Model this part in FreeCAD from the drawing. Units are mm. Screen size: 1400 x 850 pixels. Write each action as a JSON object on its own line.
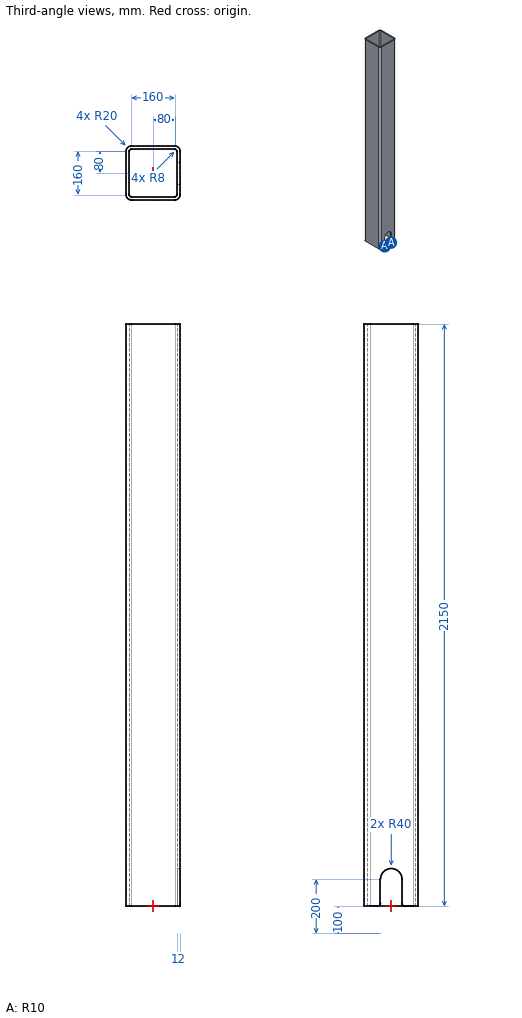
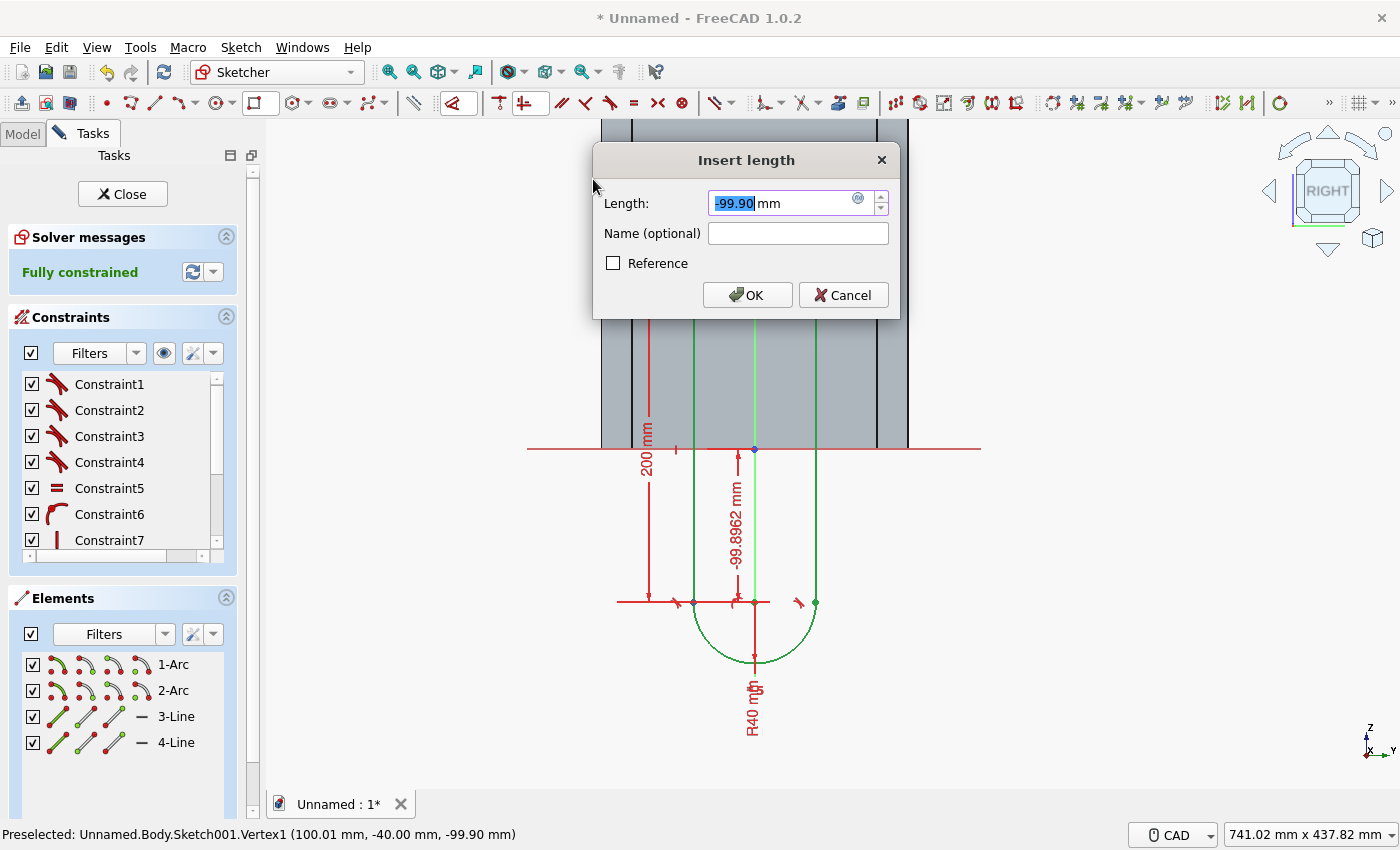
{"action": "type", "text": "-100"}
{"action": "key", "text": "Return"}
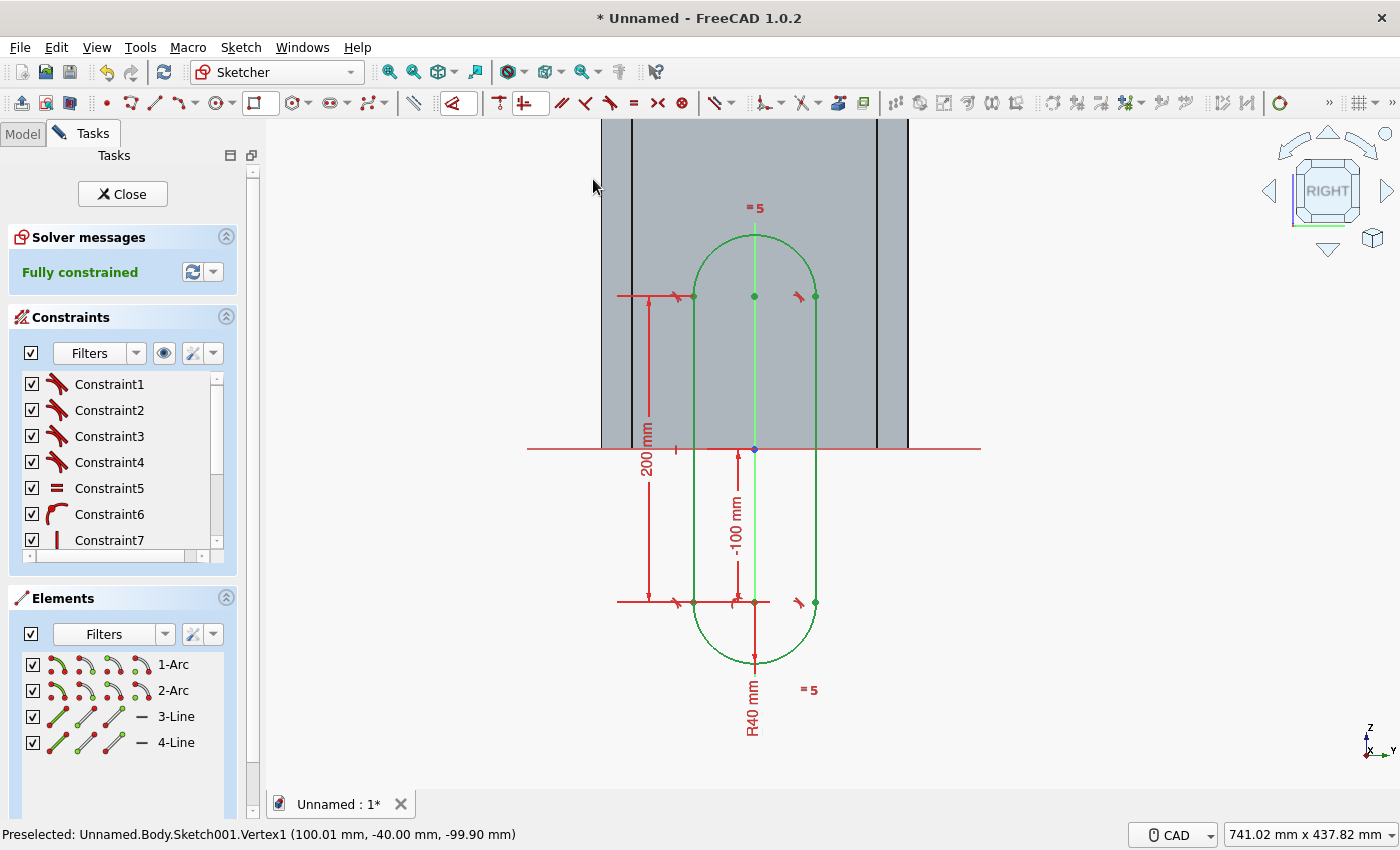
{"action": "left_click", "coordinate": [123, 194]}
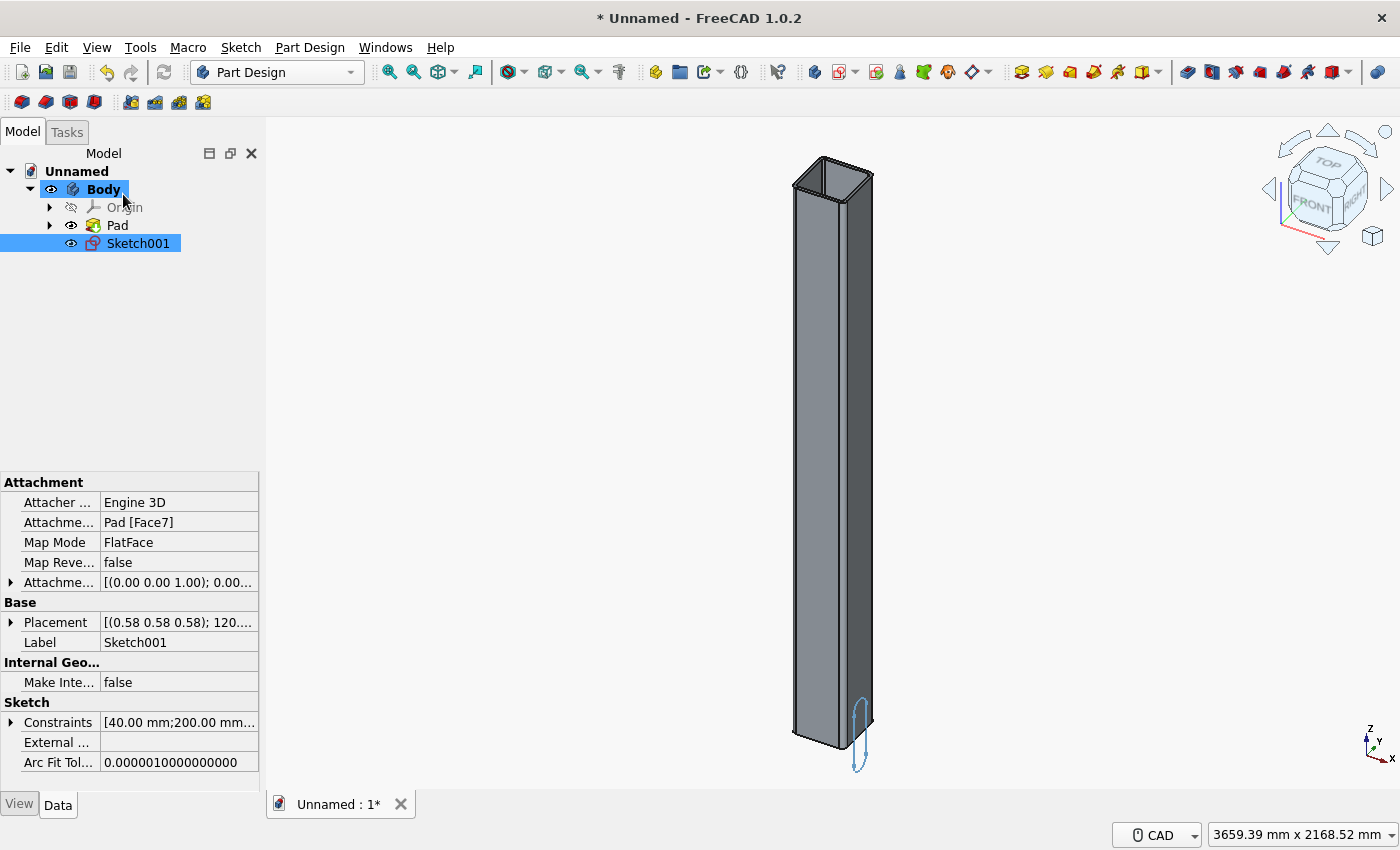
{"action": "left_click", "coordinate": [1188, 72]}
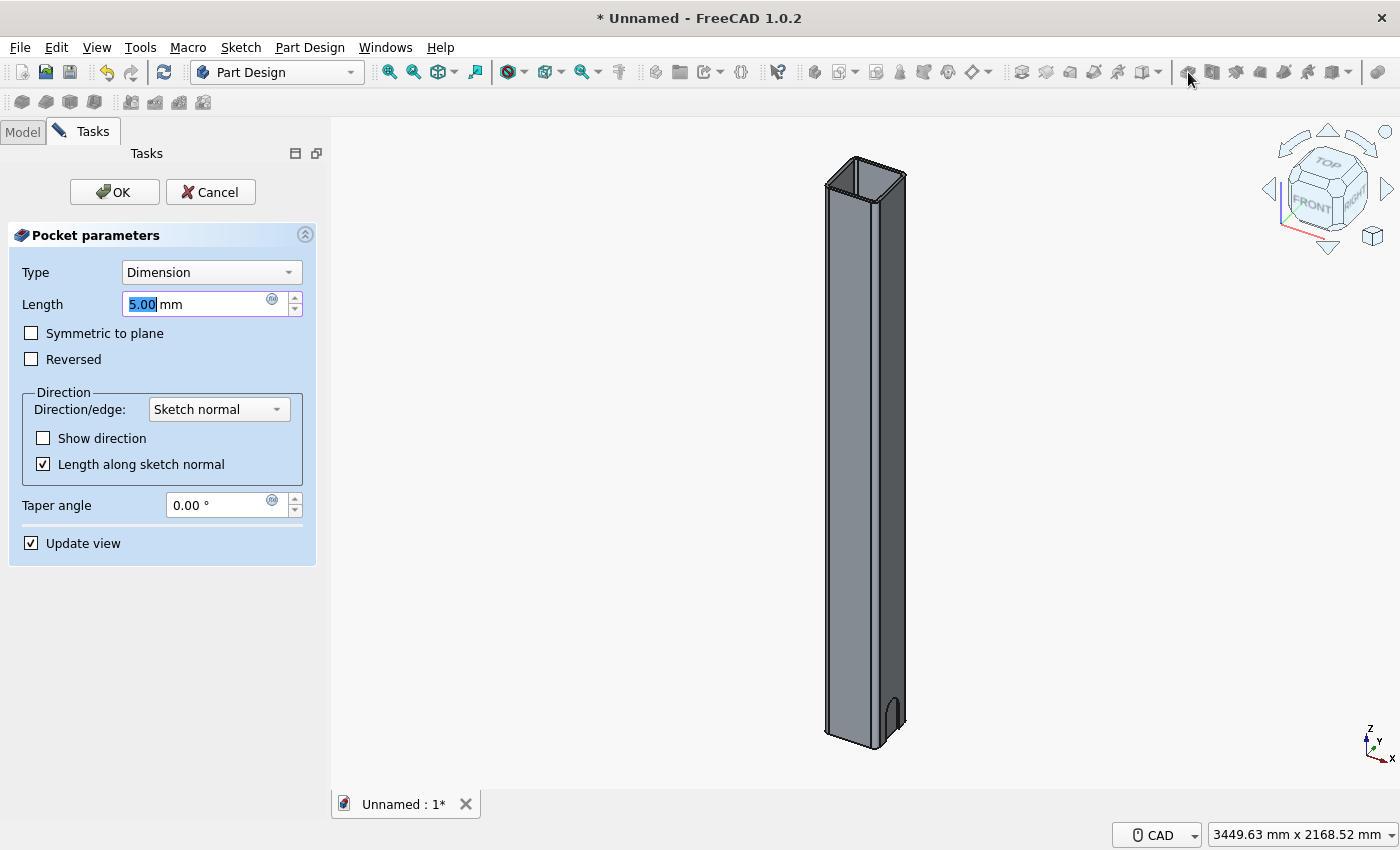
{"action": "type", "text": "12"}
{"action": "key", "text": "Tab"}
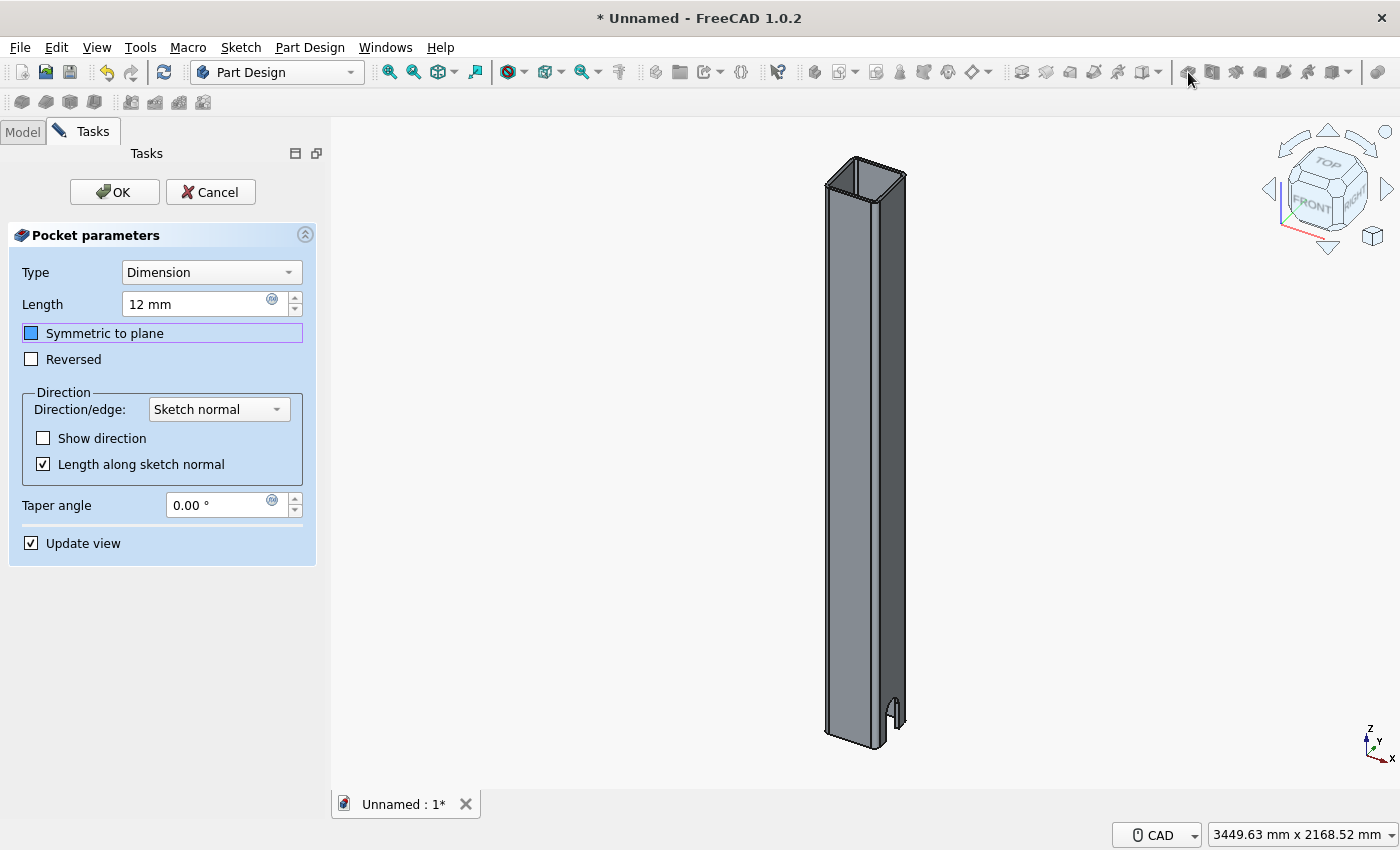
{"action": "left_click", "coordinate": [115, 192]}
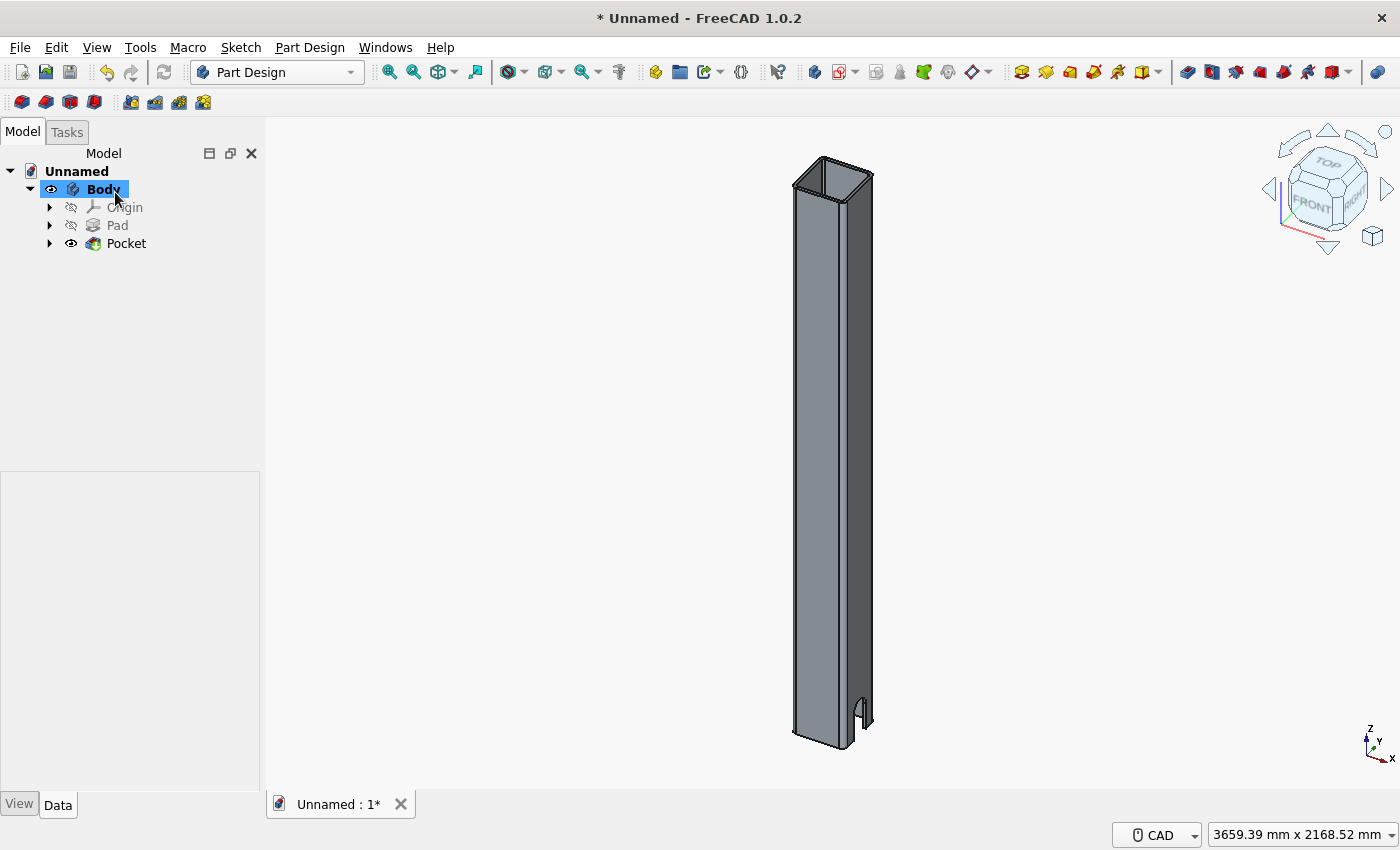
{"action": "scroll", "coordinate": [852, 739], "scroll_direction": "up", "scroll_amount": 12}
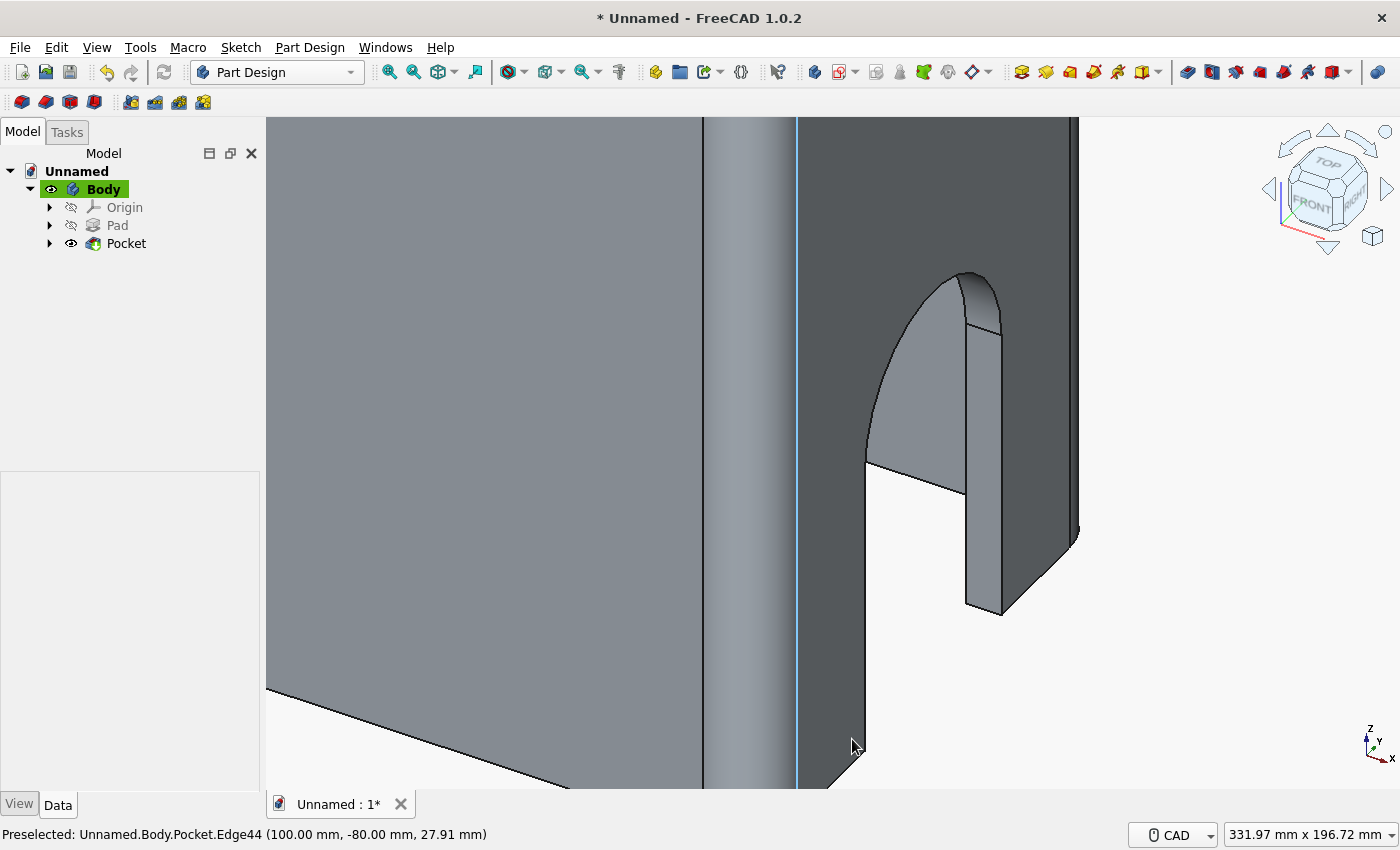
{"action": "left_click", "coordinate": [390, 72]}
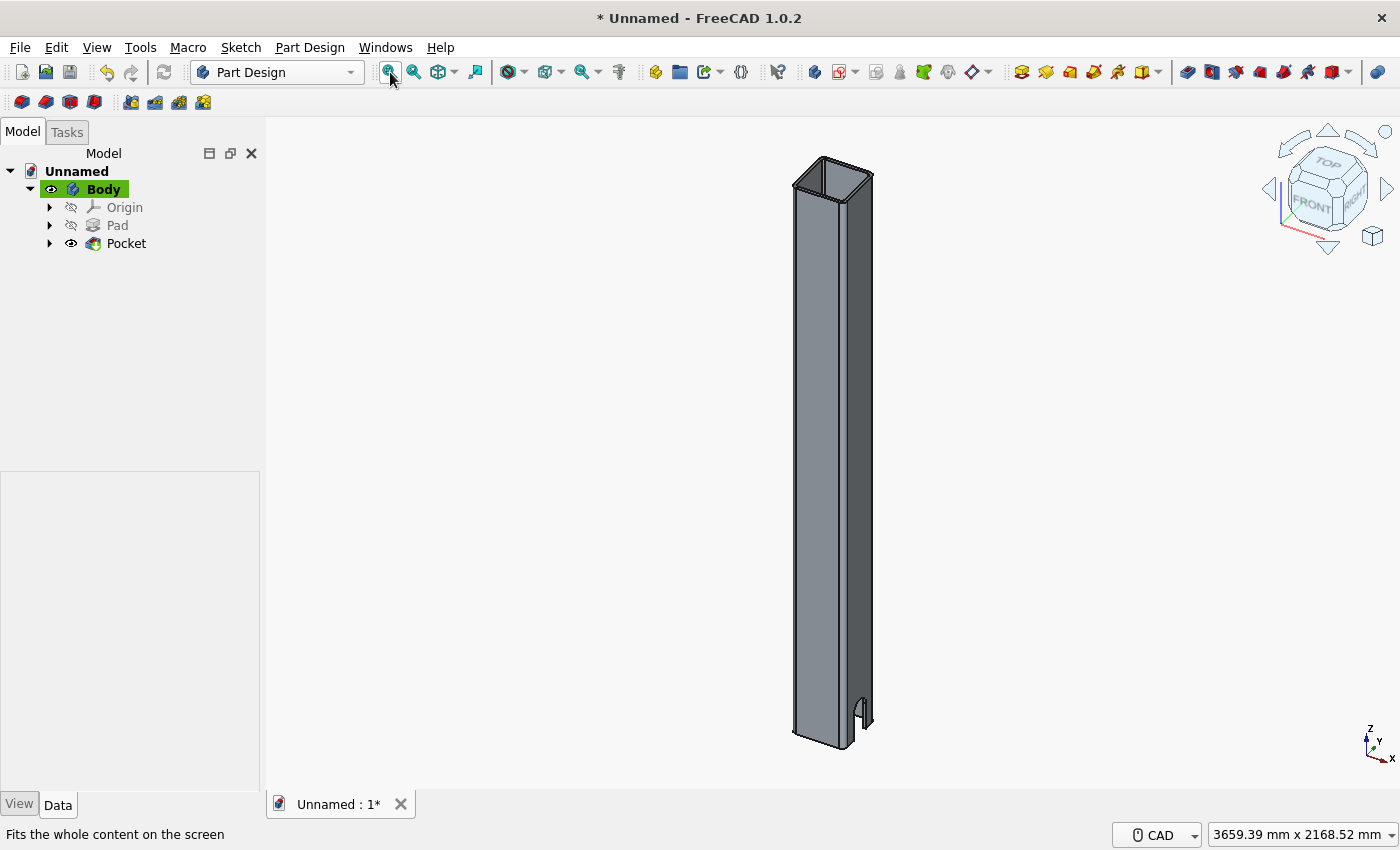
{"action": "key", "text": "0"}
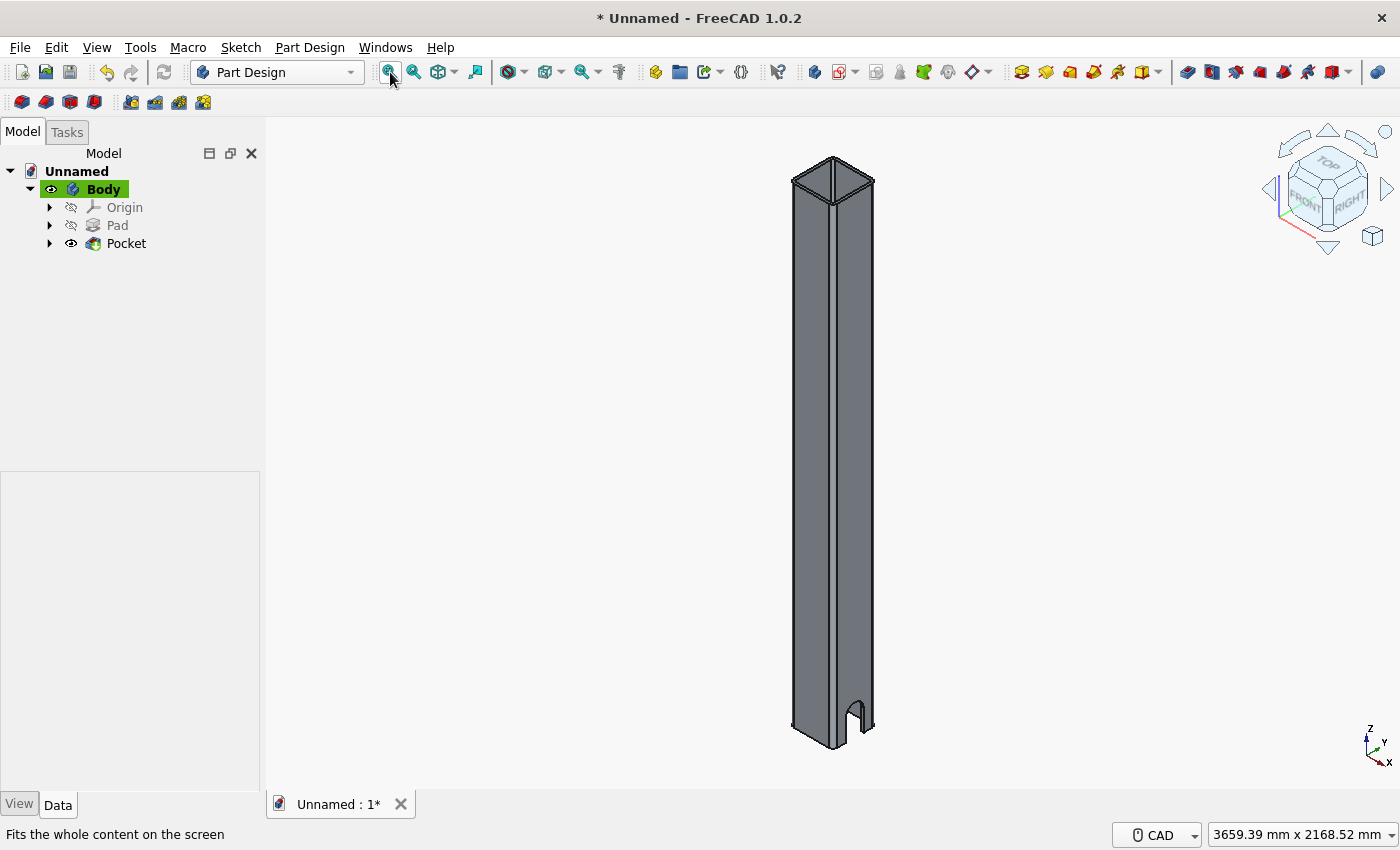
{"action": "scroll", "coordinate": [845, 741], "scroll_direction": "up", "scroll_amount": 12}